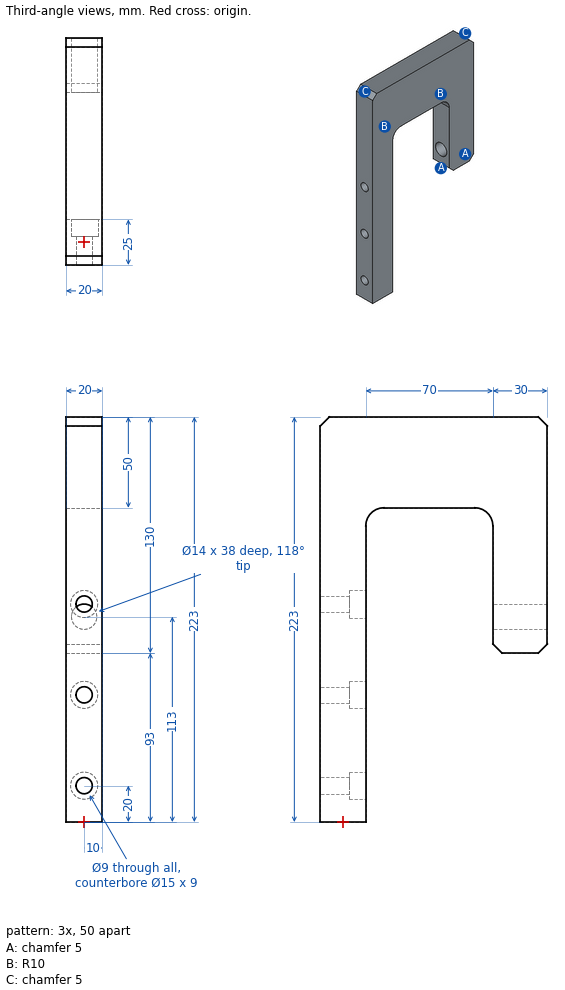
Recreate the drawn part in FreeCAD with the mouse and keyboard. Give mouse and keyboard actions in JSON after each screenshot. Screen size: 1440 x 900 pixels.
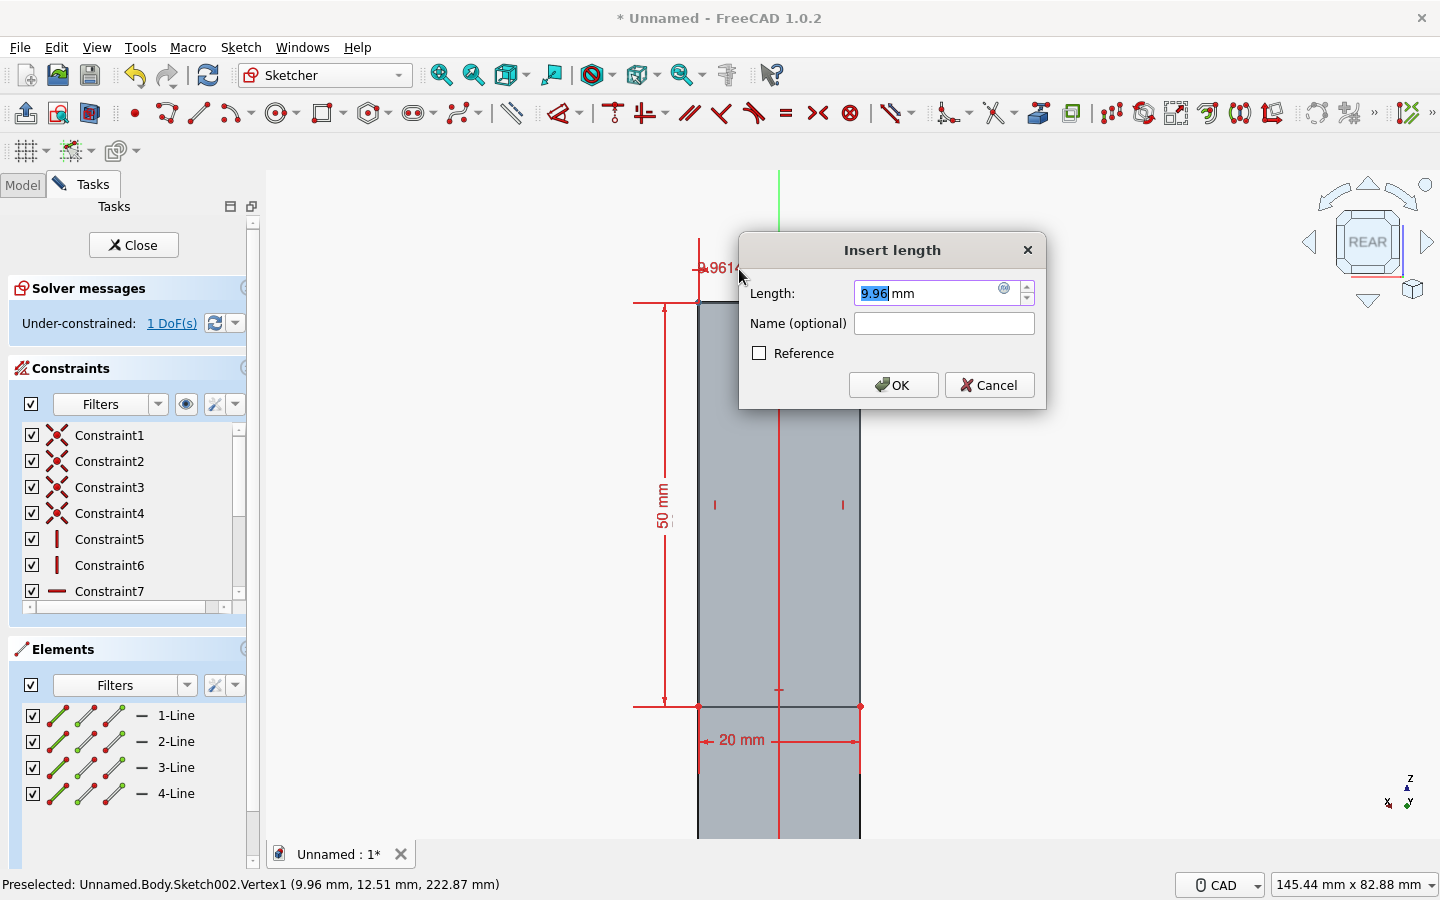
{"action": "type", "text": "10"}
{"action": "key", "text": "Return"}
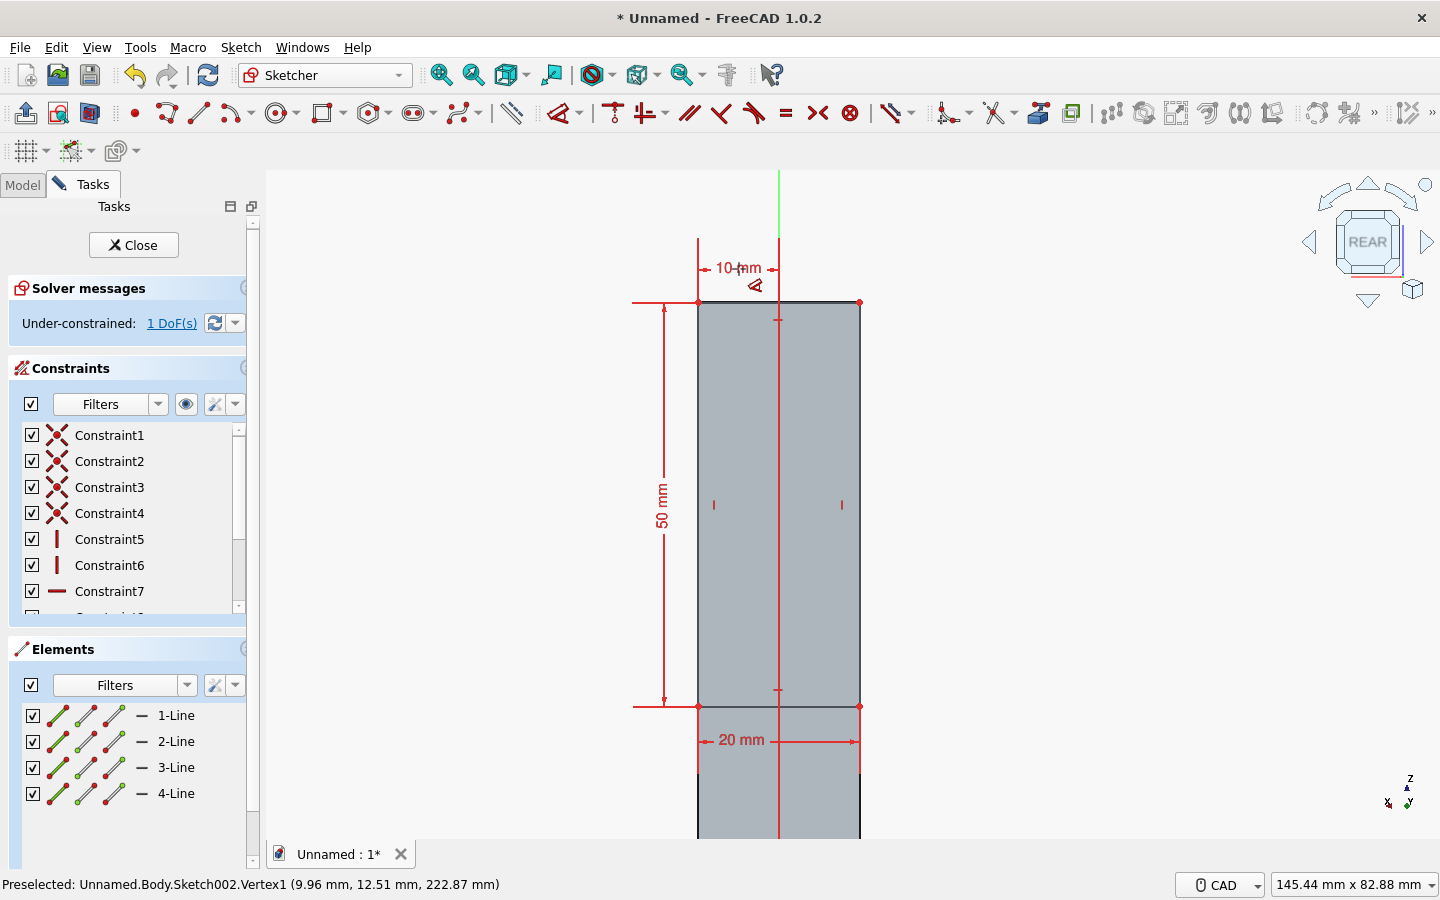
{"action": "left_click", "coordinate": [698, 303]}
{"action": "left_click", "coordinate": [664, 557]}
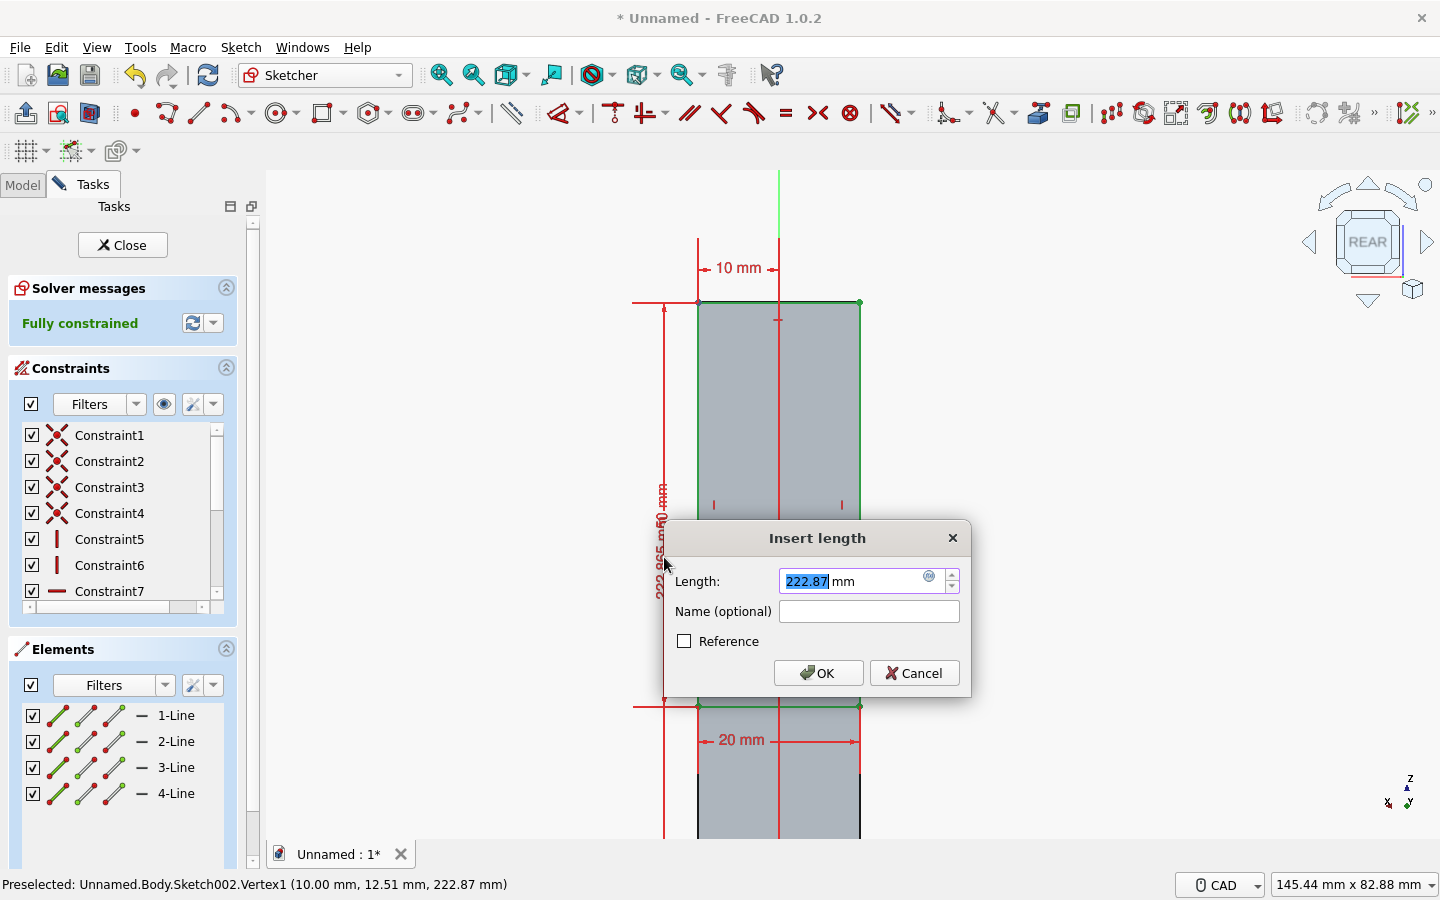
{"action": "type", "text": "223"}
{"action": "key", "text": "Return"}
{"action": "key", "text": "Escape"}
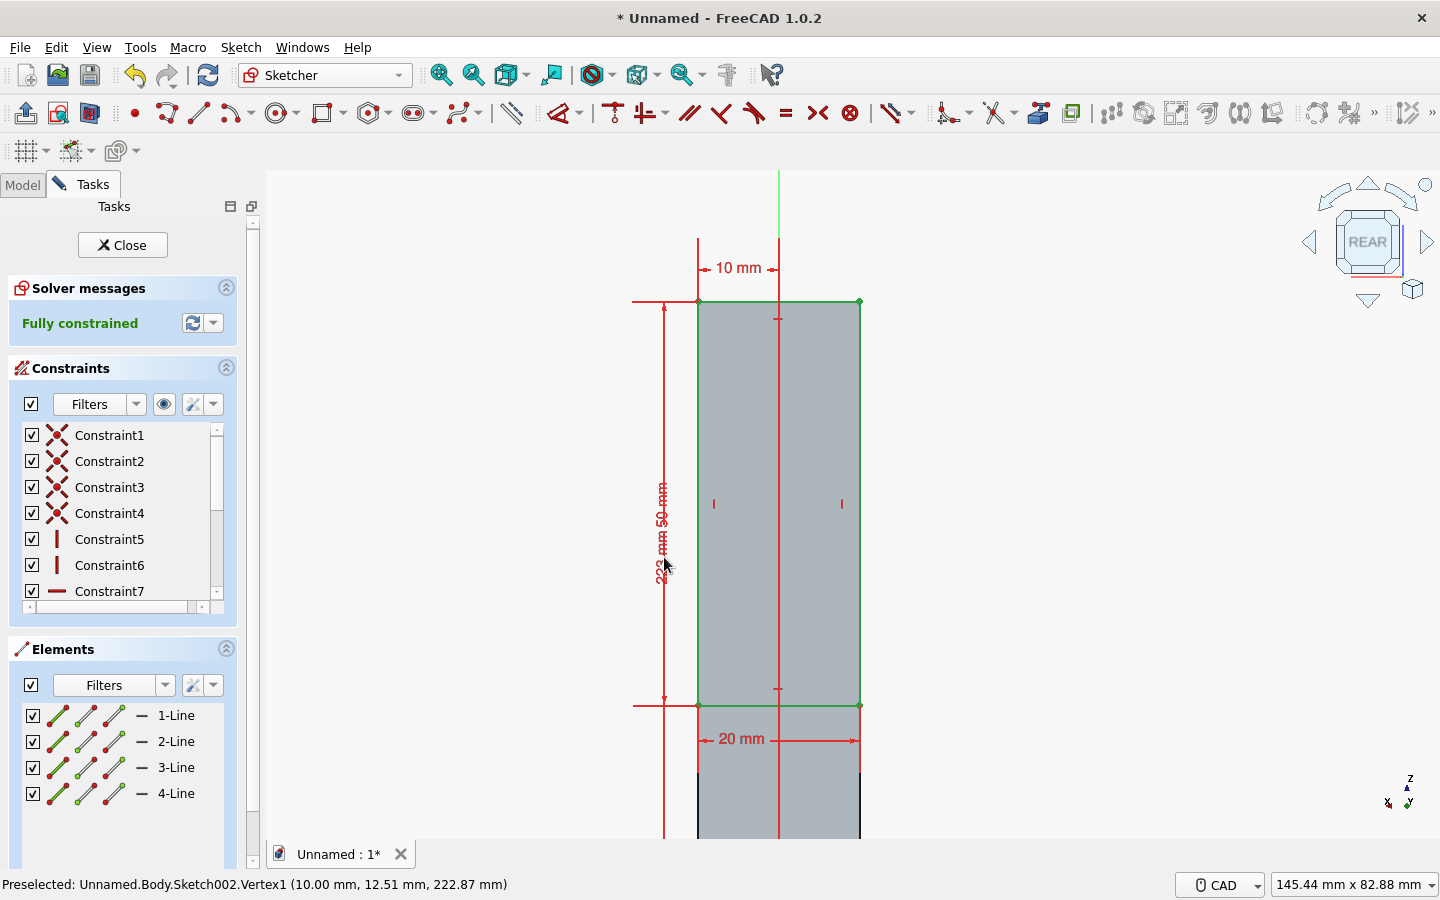
{"action": "left_click", "coordinate": [123, 245]}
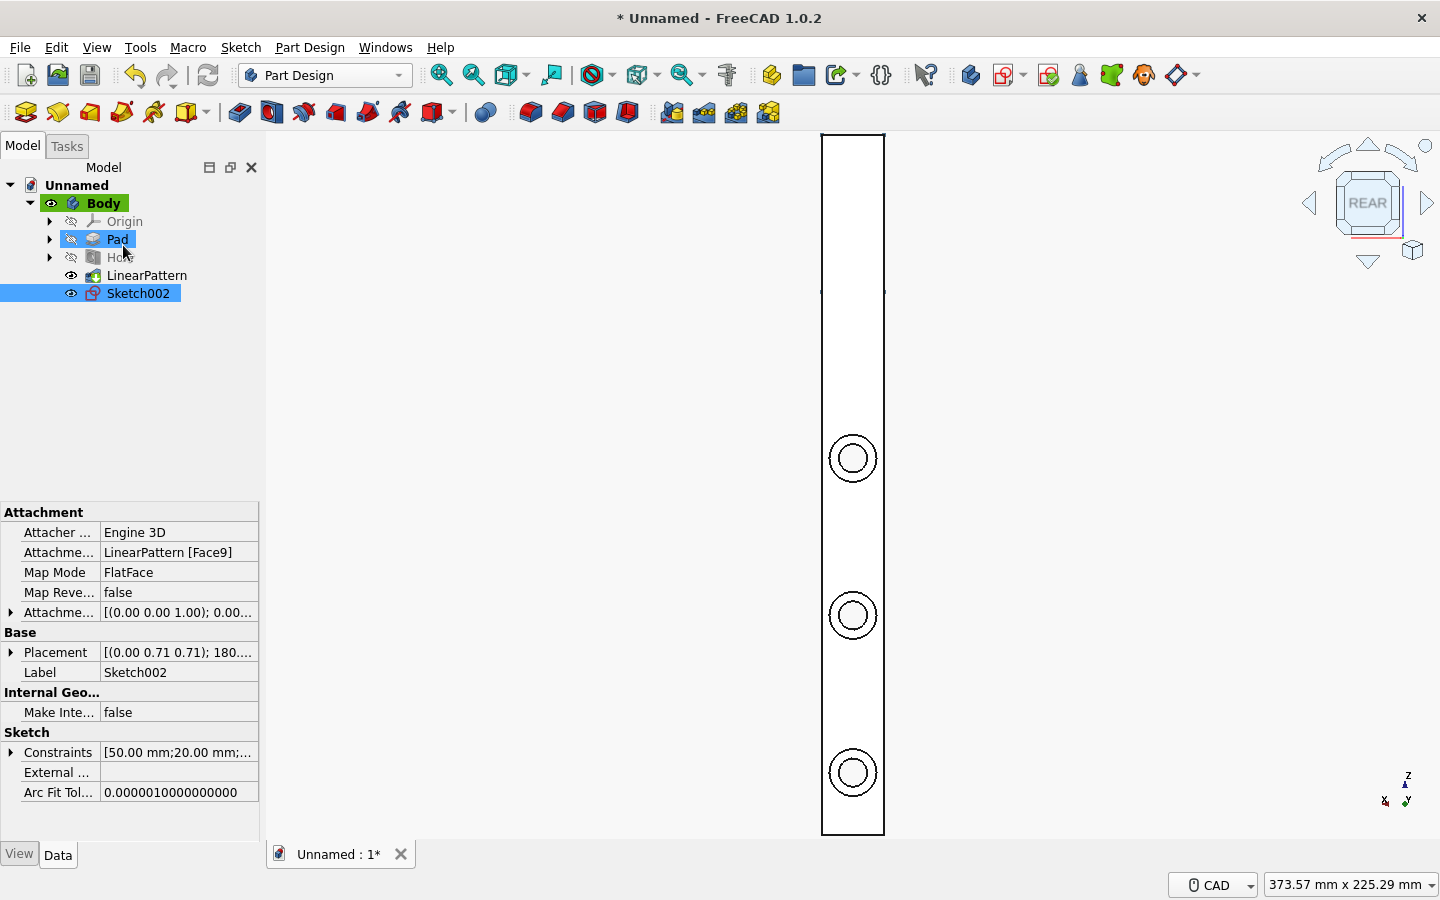
{"action": "left_click", "coordinate": [26, 112]}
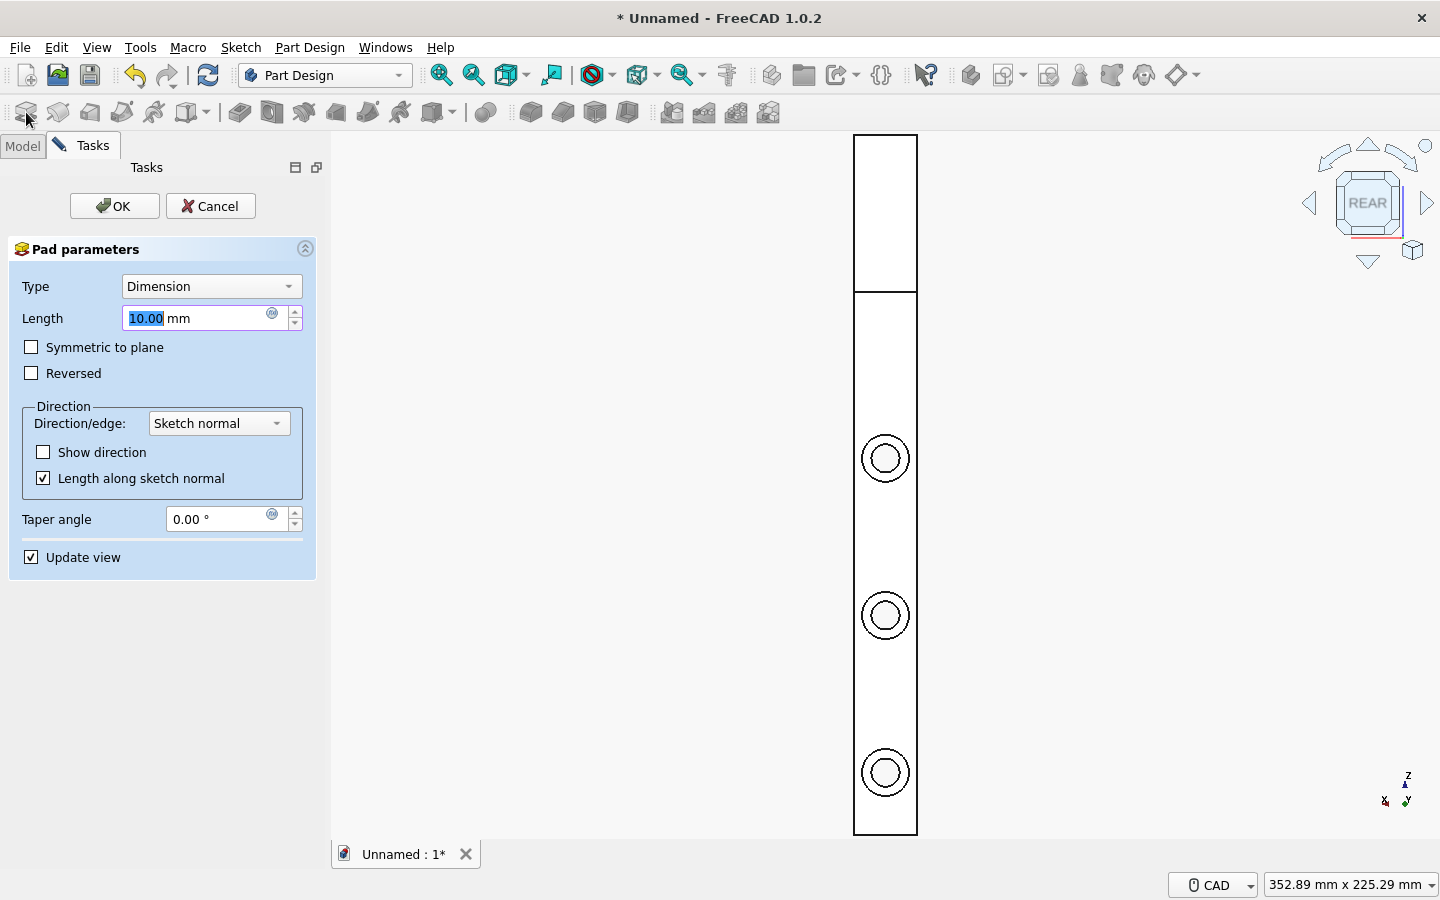
{"action": "type", "text": "70"}
{"action": "key", "text": "Tab"}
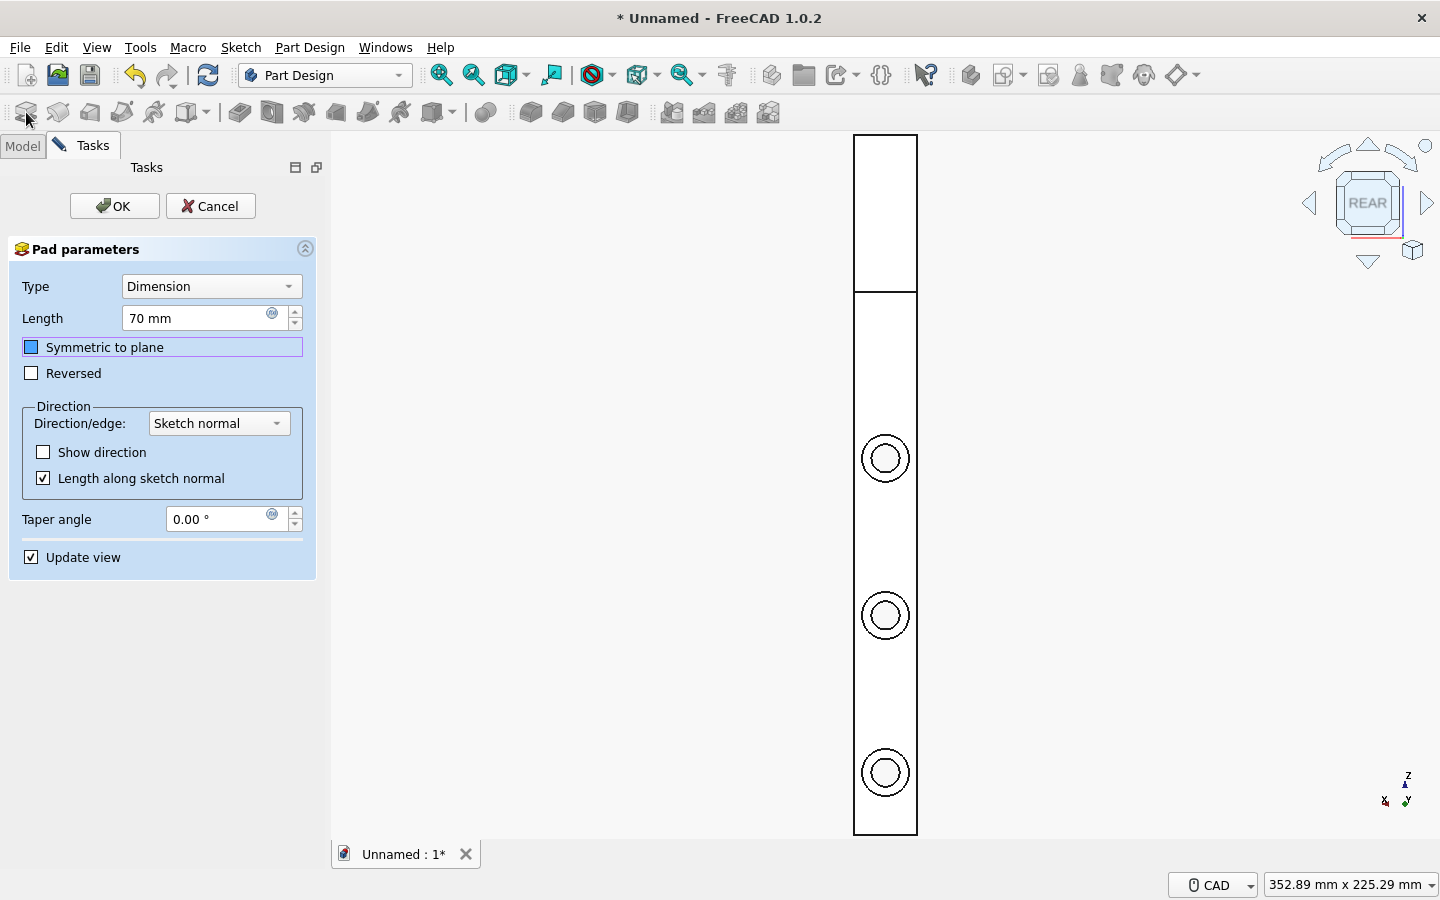
{"action": "left_click", "coordinate": [115, 206]}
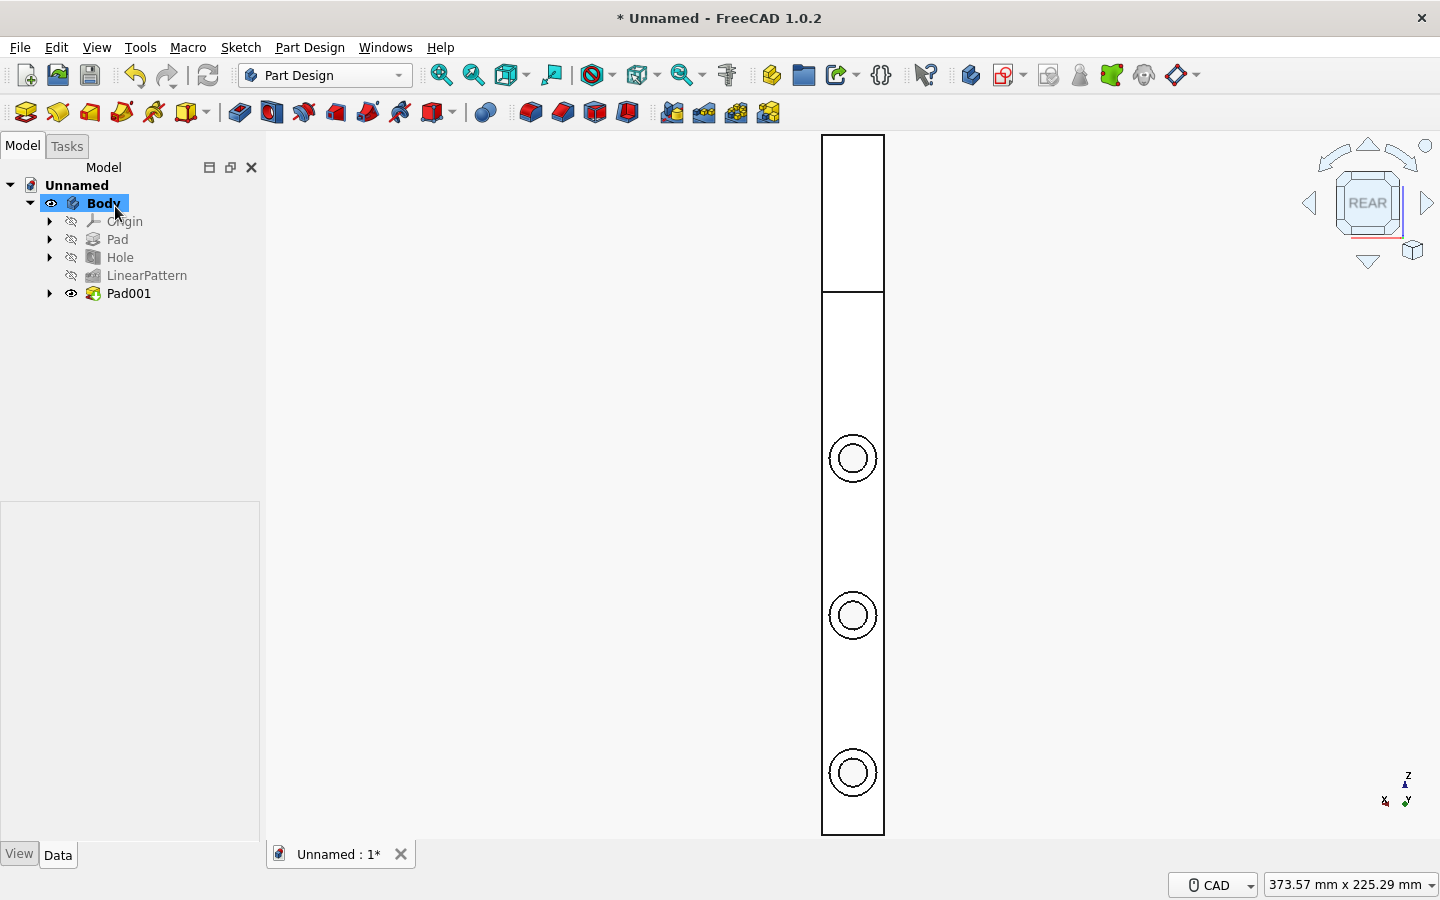
{"action": "left_click", "coordinate": [853, 167]}